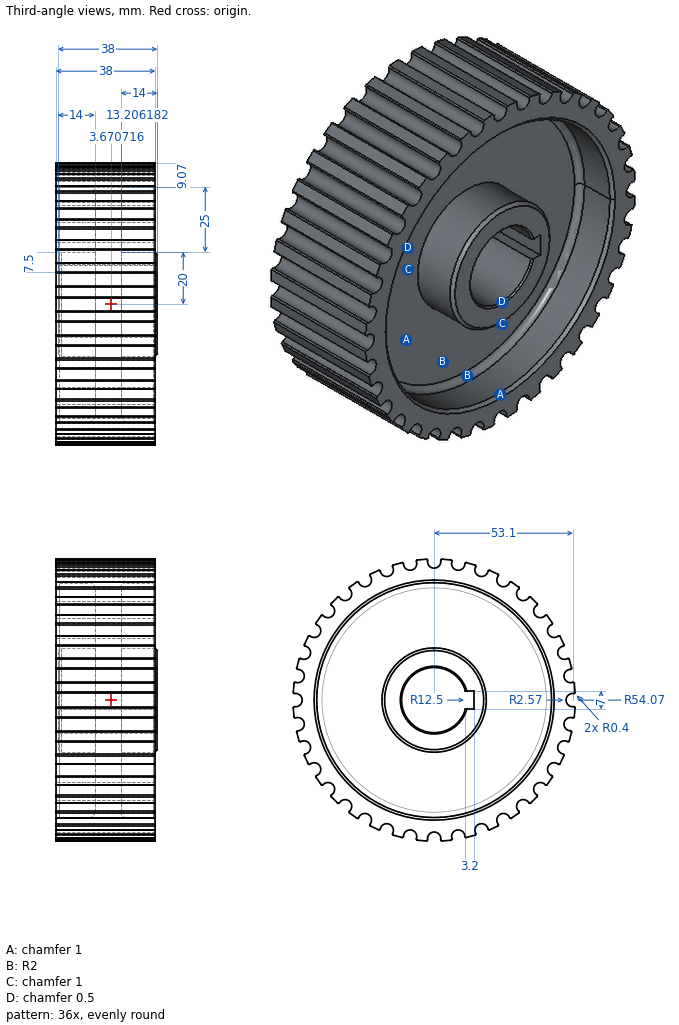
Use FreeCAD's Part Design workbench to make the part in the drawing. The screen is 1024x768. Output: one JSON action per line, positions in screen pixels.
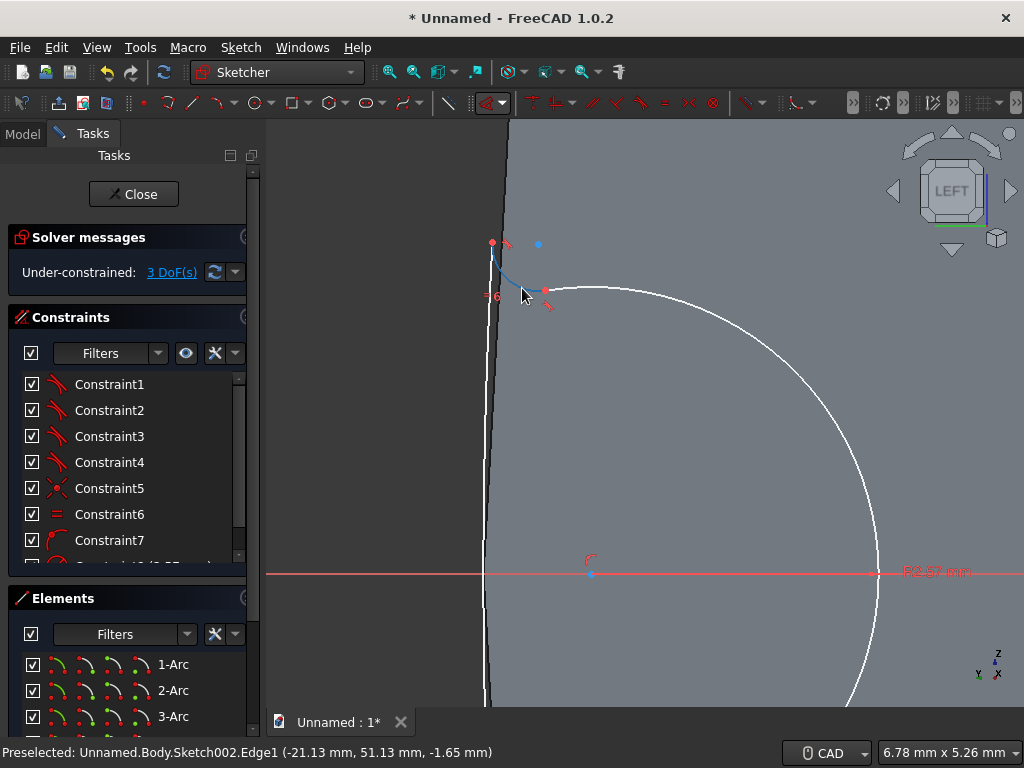
{"action": "left_click", "coordinate": [522, 288]}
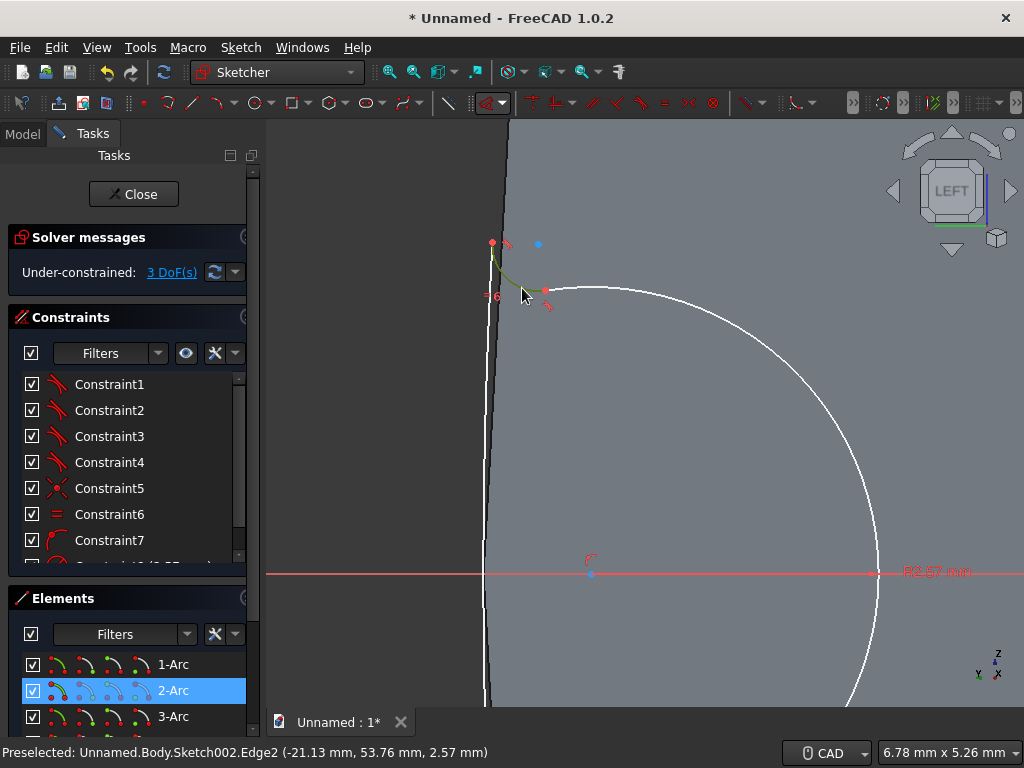
{"action": "key", "text": "k r"}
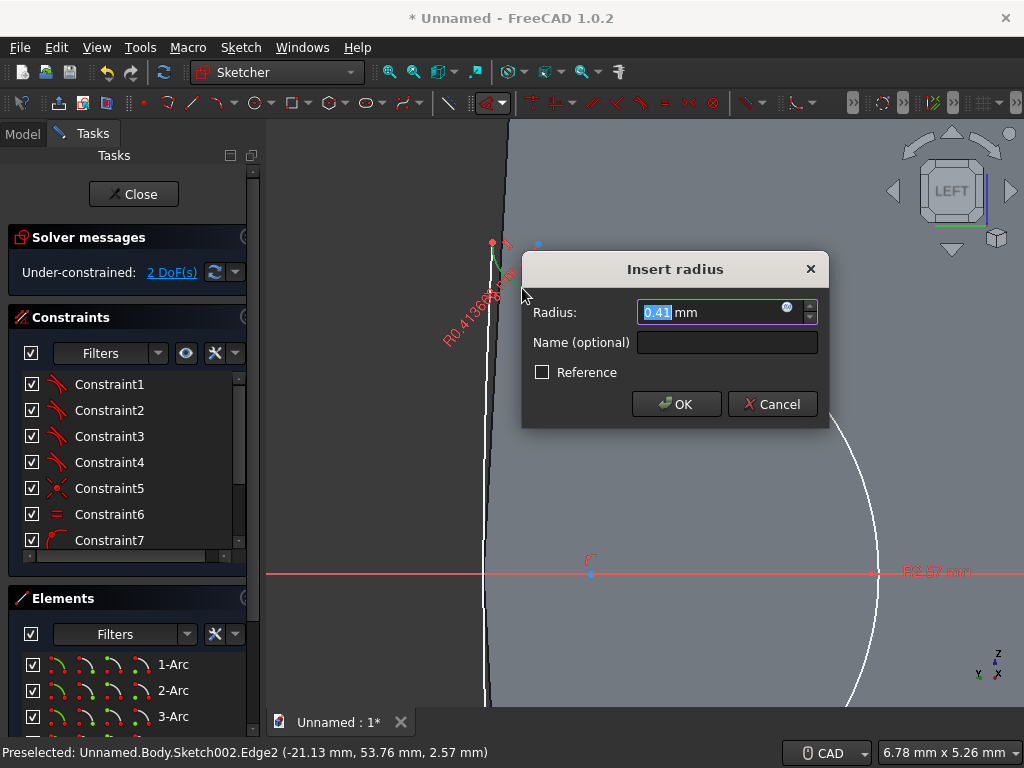
{"action": "type", "text": "0.4"}
{"action": "key", "text": "Return"}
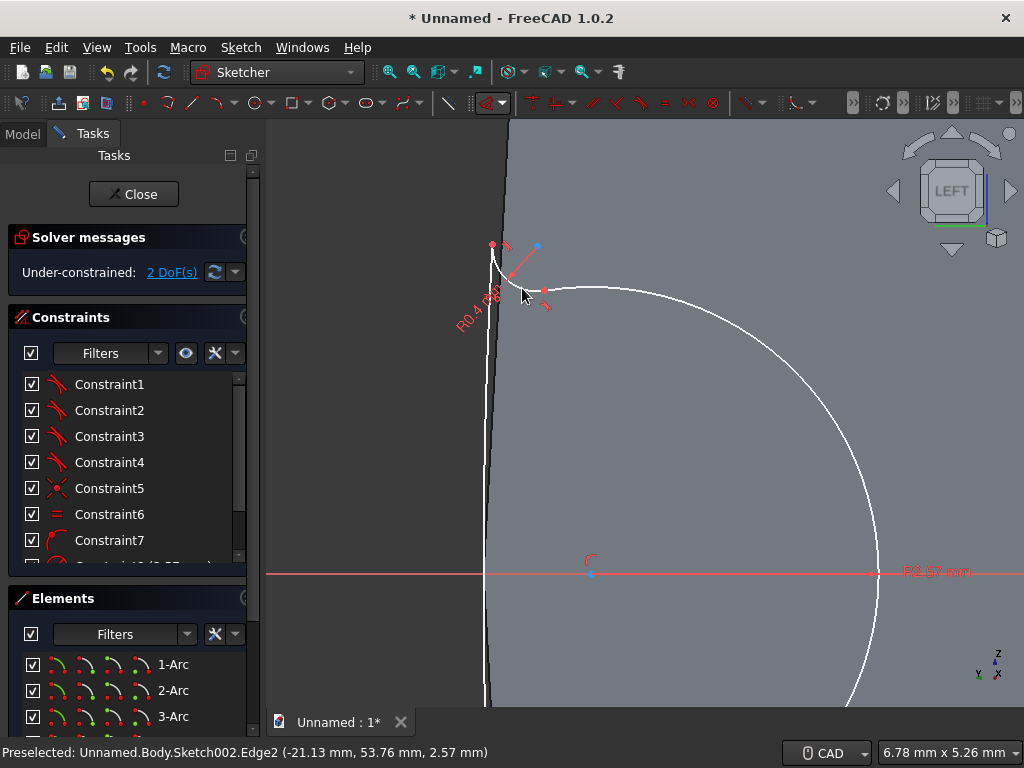
{"action": "left_click", "coordinate": [485, 442]}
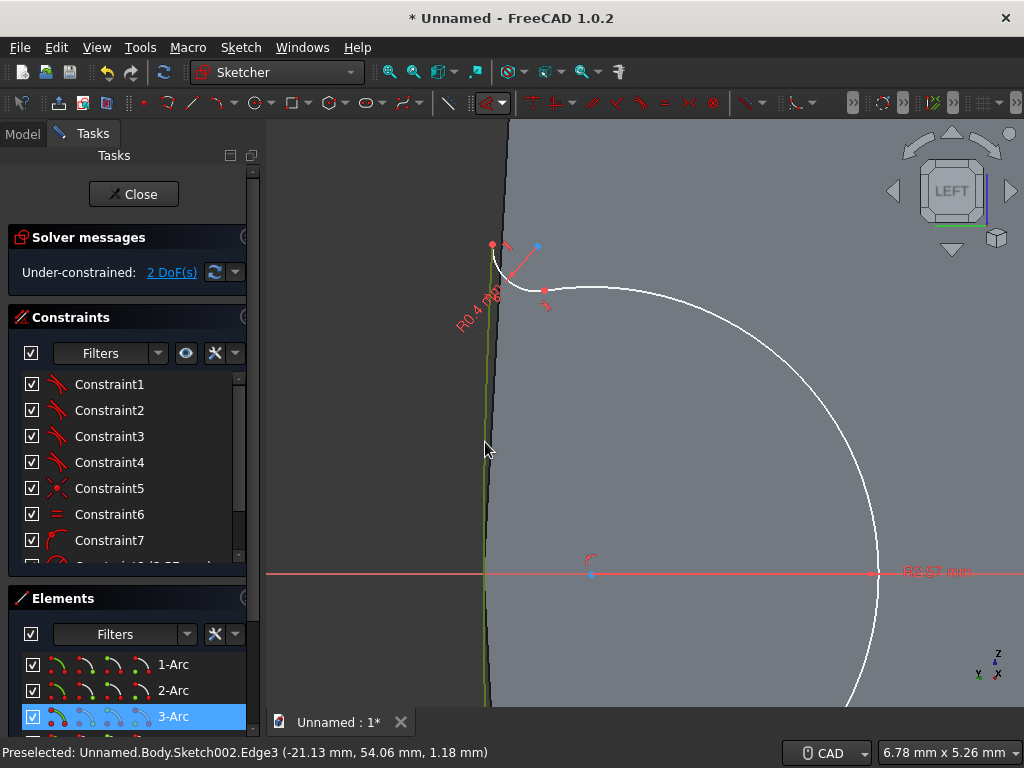
{"action": "key", "text": "k r"}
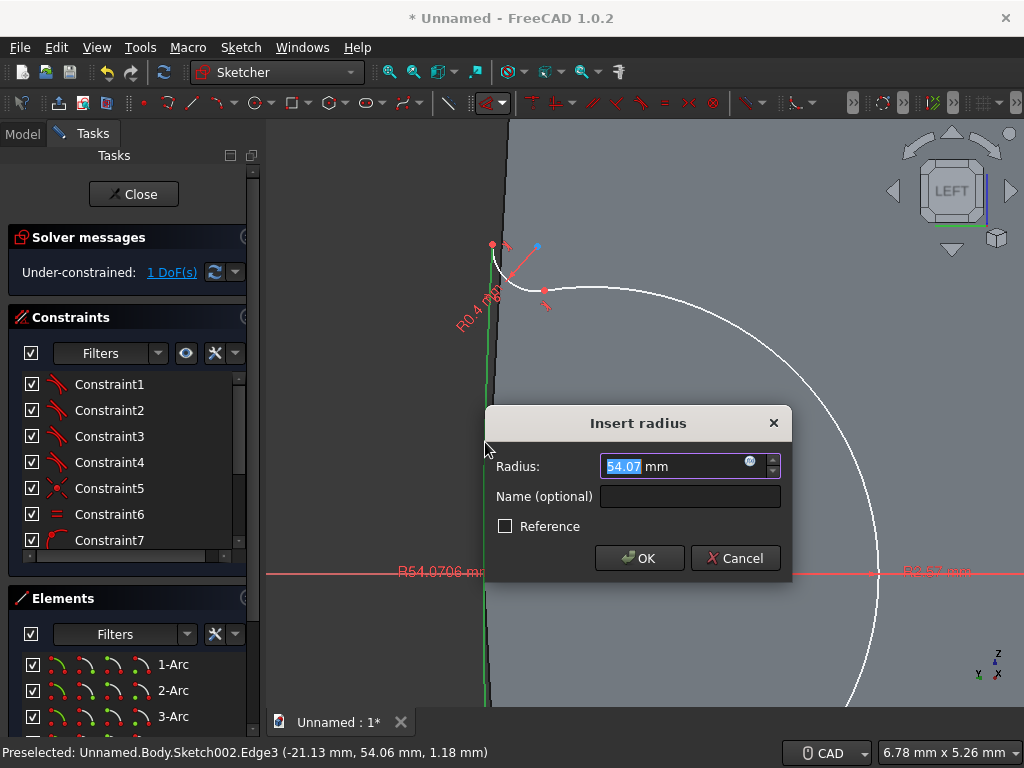
{"action": "type", "text": "54.07"}
{"action": "key", "text": "Return"}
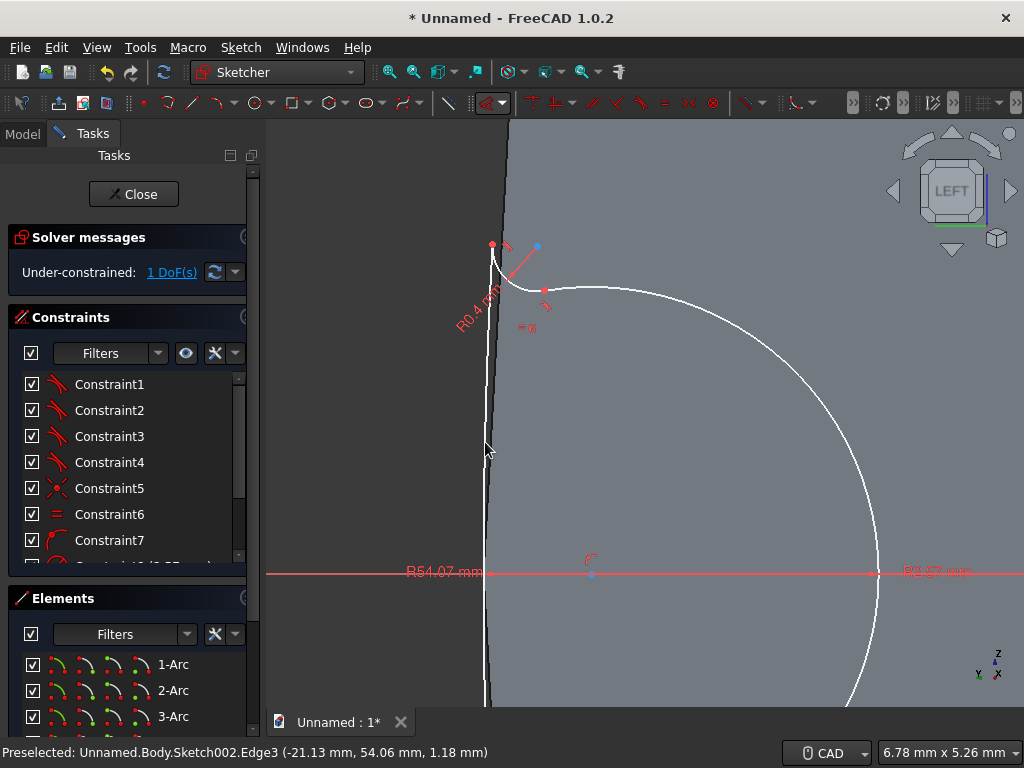
{"action": "left_click", "coordinate": [592, 574]}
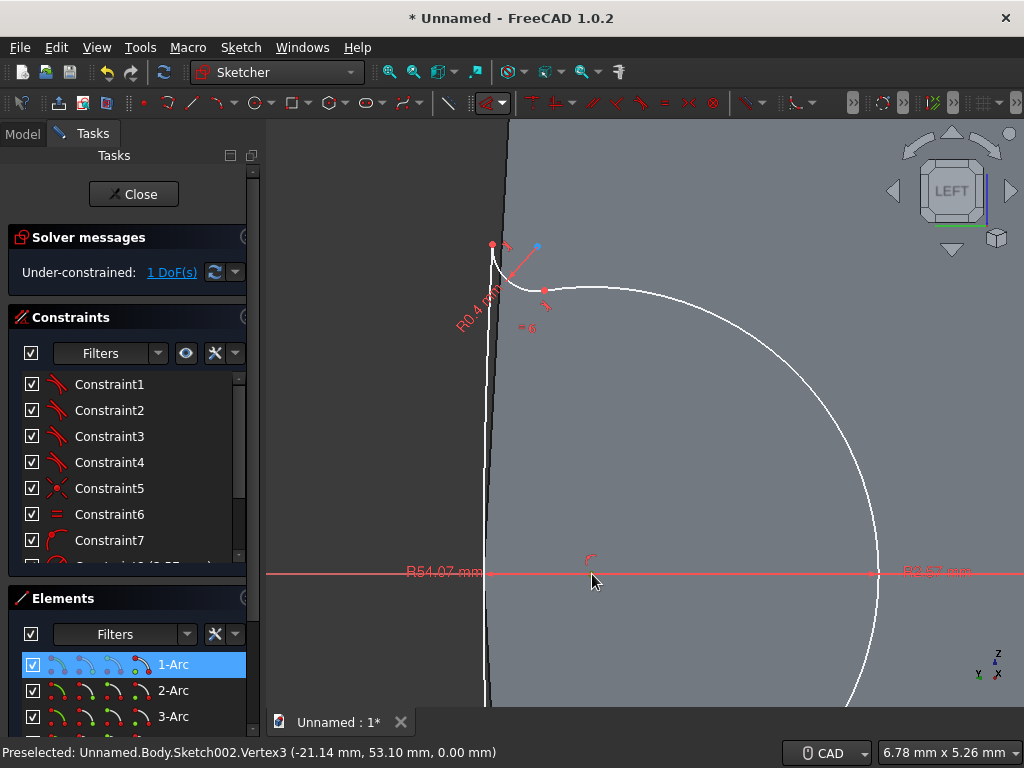
{"action": "left_click", "coordinate": [504, 104]}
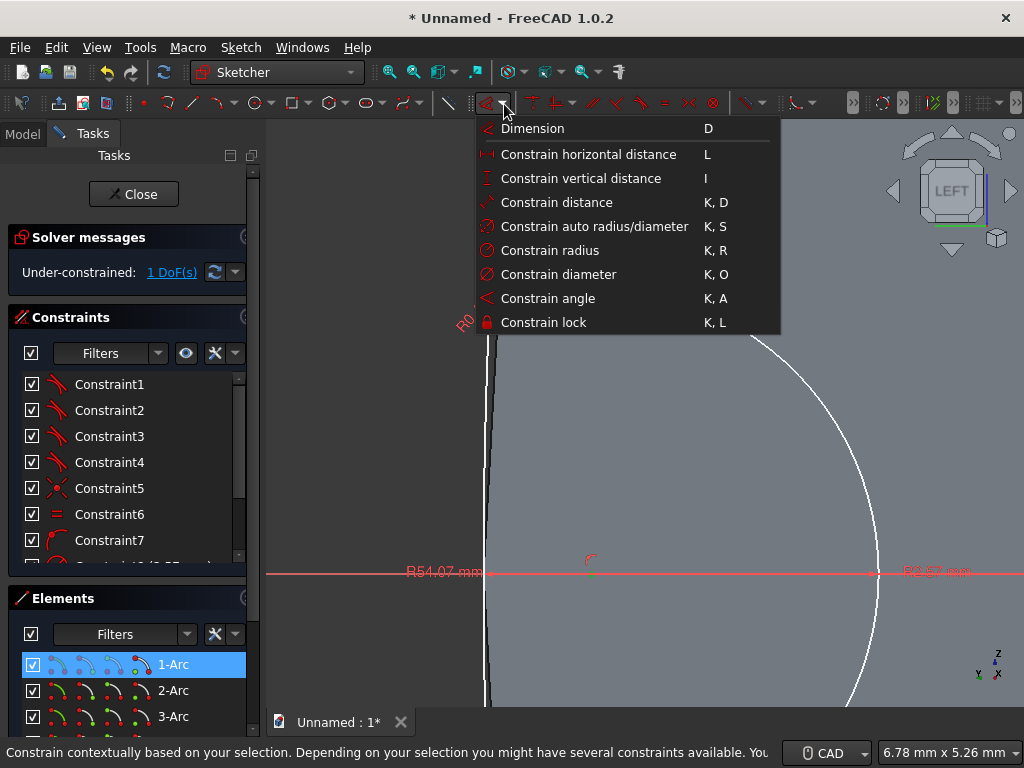
{"action": "left_click", "coordinate": [628, 154]}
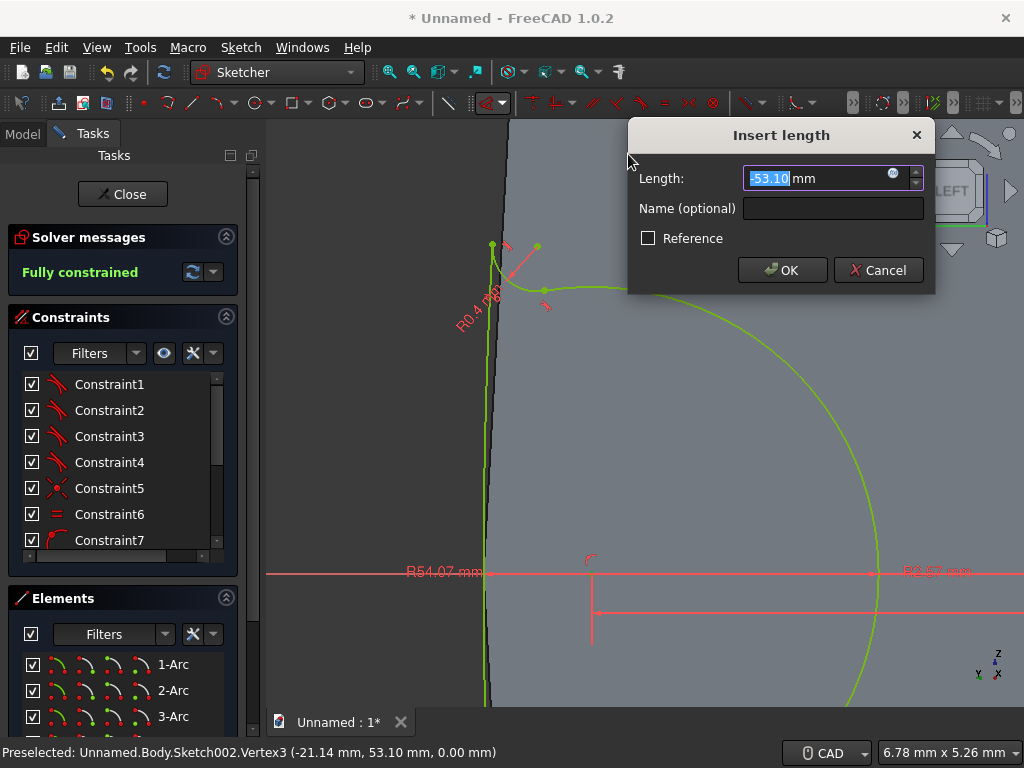
{"action": "type", "text": "-53.1"}
{"action": "key", "text": "Return"}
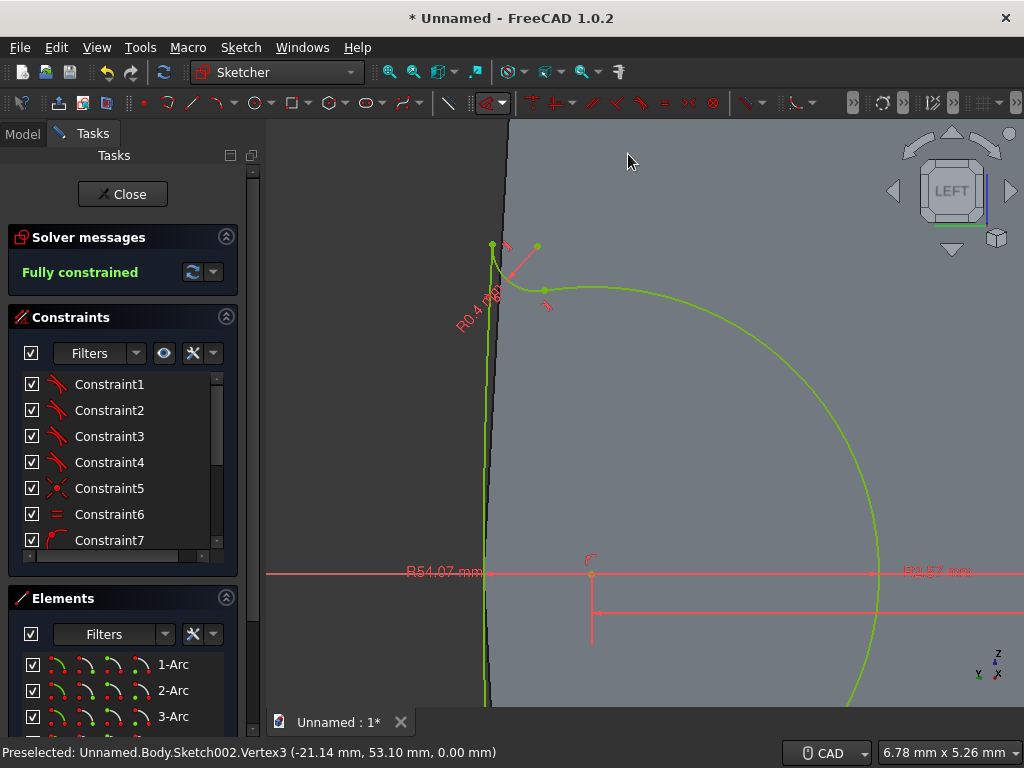
{"action": "left_click", "coordinate": [123, 194]}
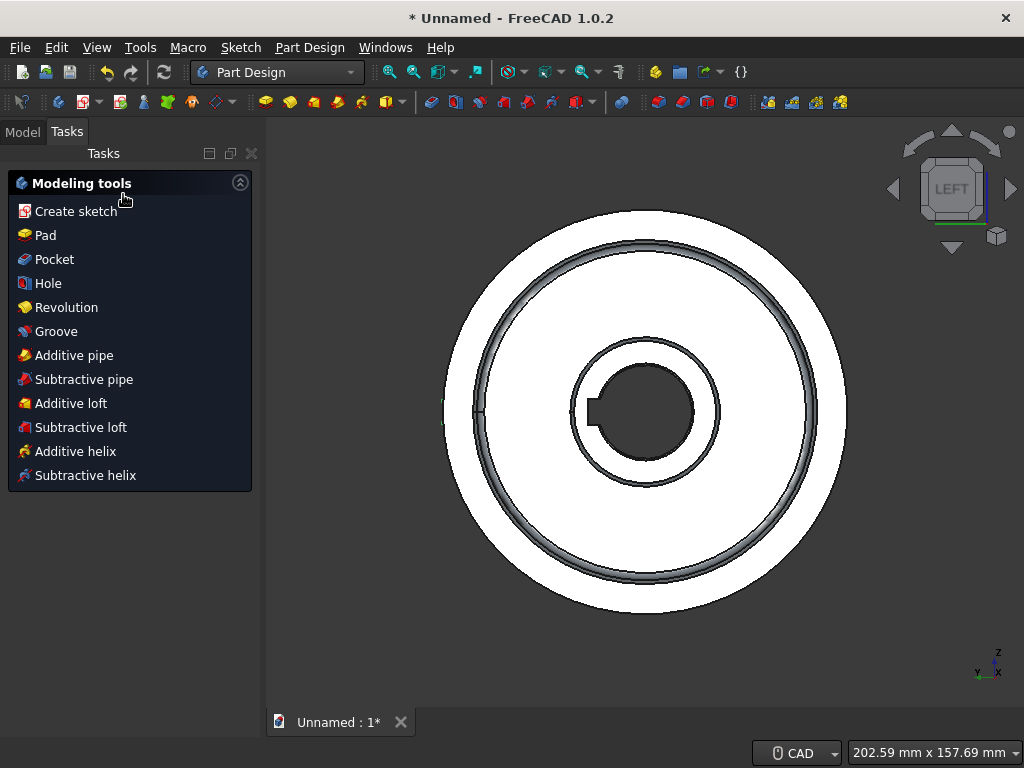
{"action": "left_click", "coordinate": [432, 102]}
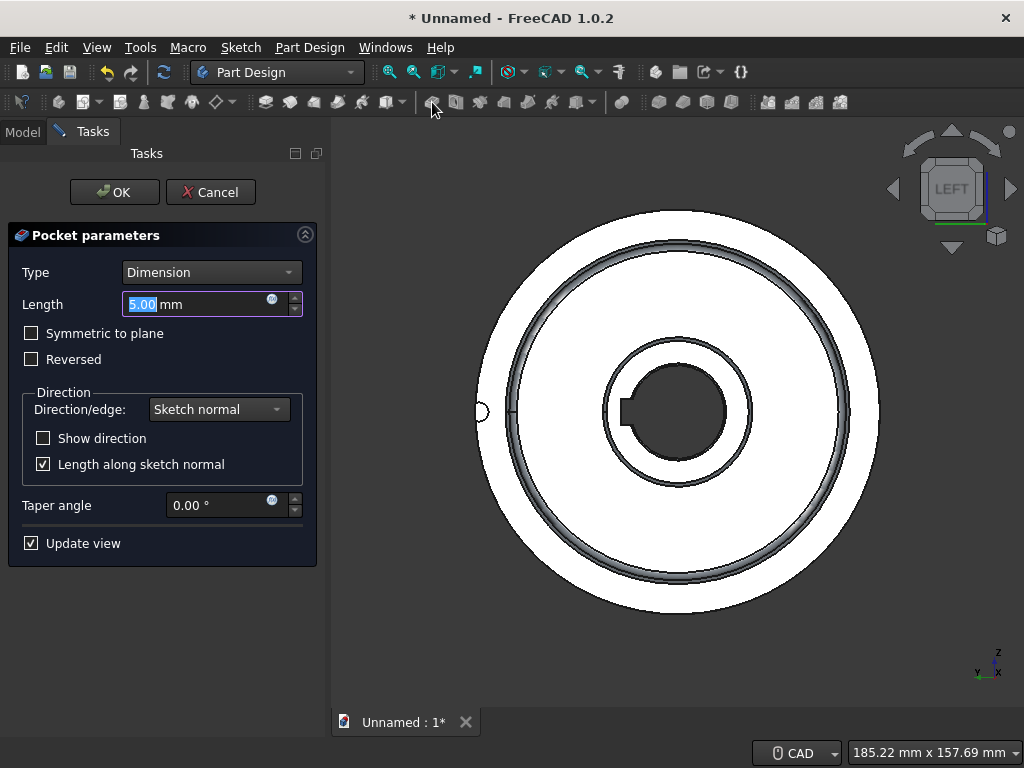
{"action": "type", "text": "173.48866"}
{"action": "key", "text": "Tab"}